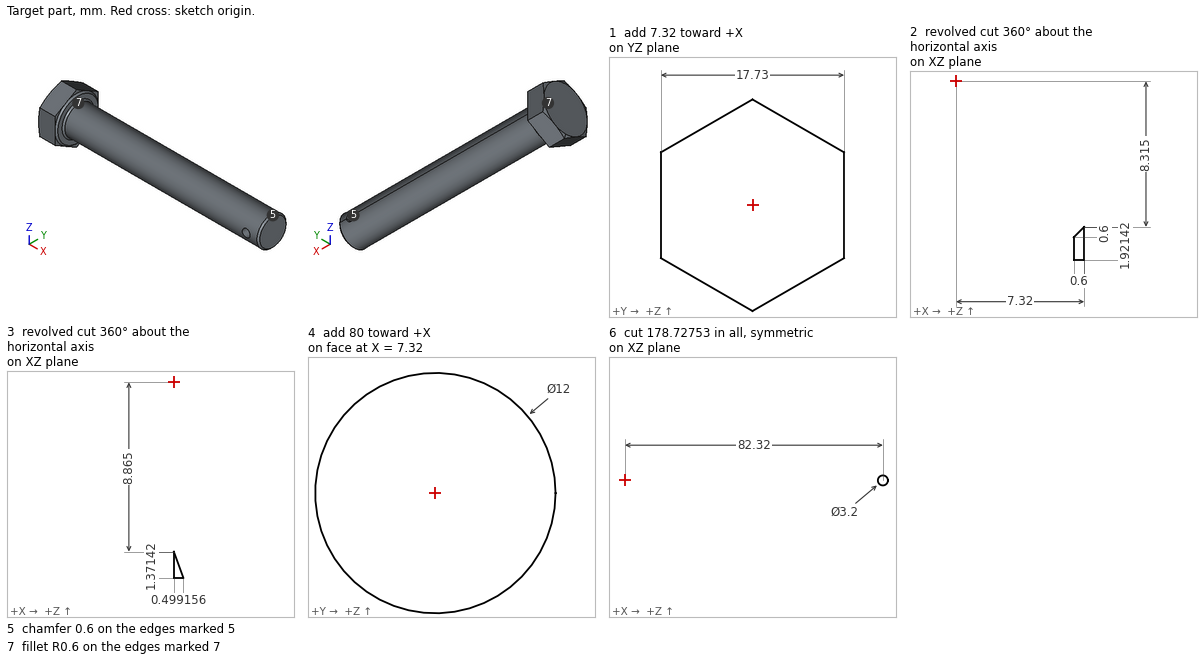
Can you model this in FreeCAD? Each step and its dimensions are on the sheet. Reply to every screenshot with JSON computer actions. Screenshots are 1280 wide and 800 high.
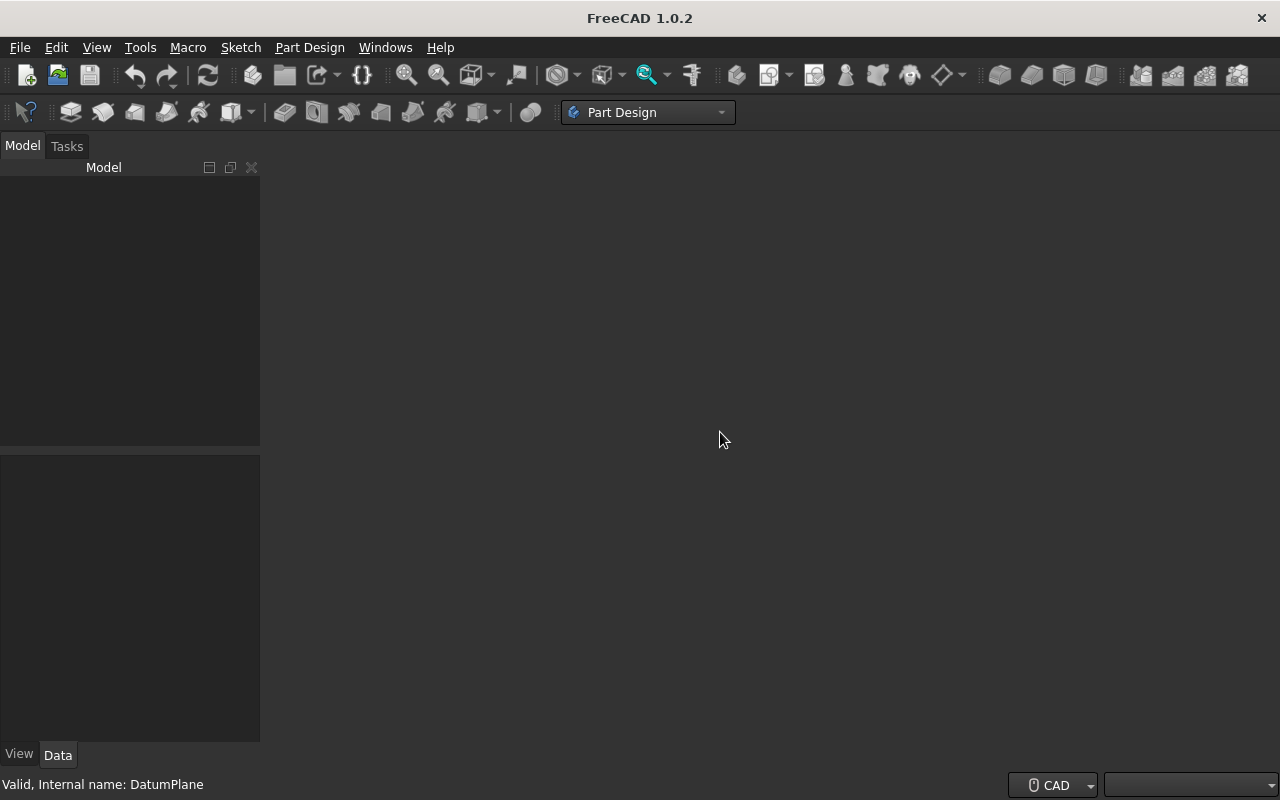
{"action": "left_click", "coordinate": [26, 76]}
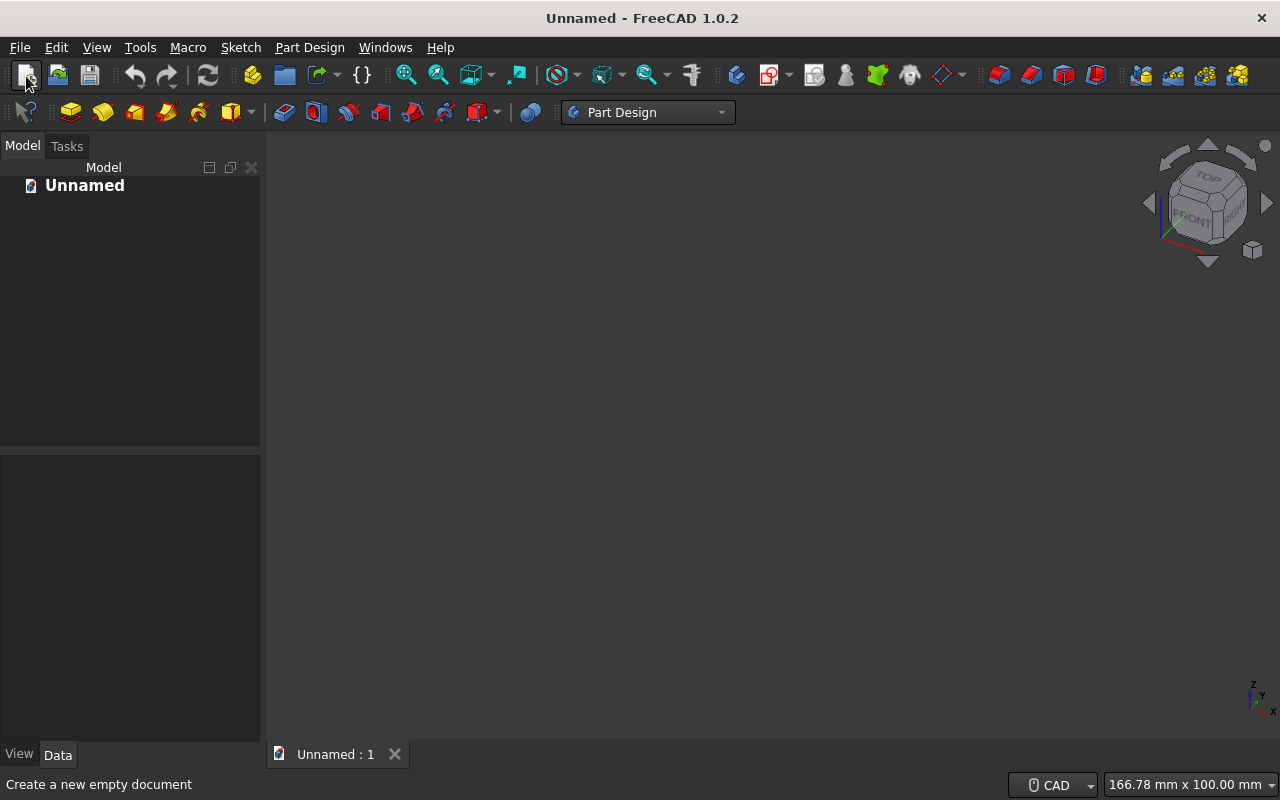
{"action": "left_click", "coordinate": [770, 76]}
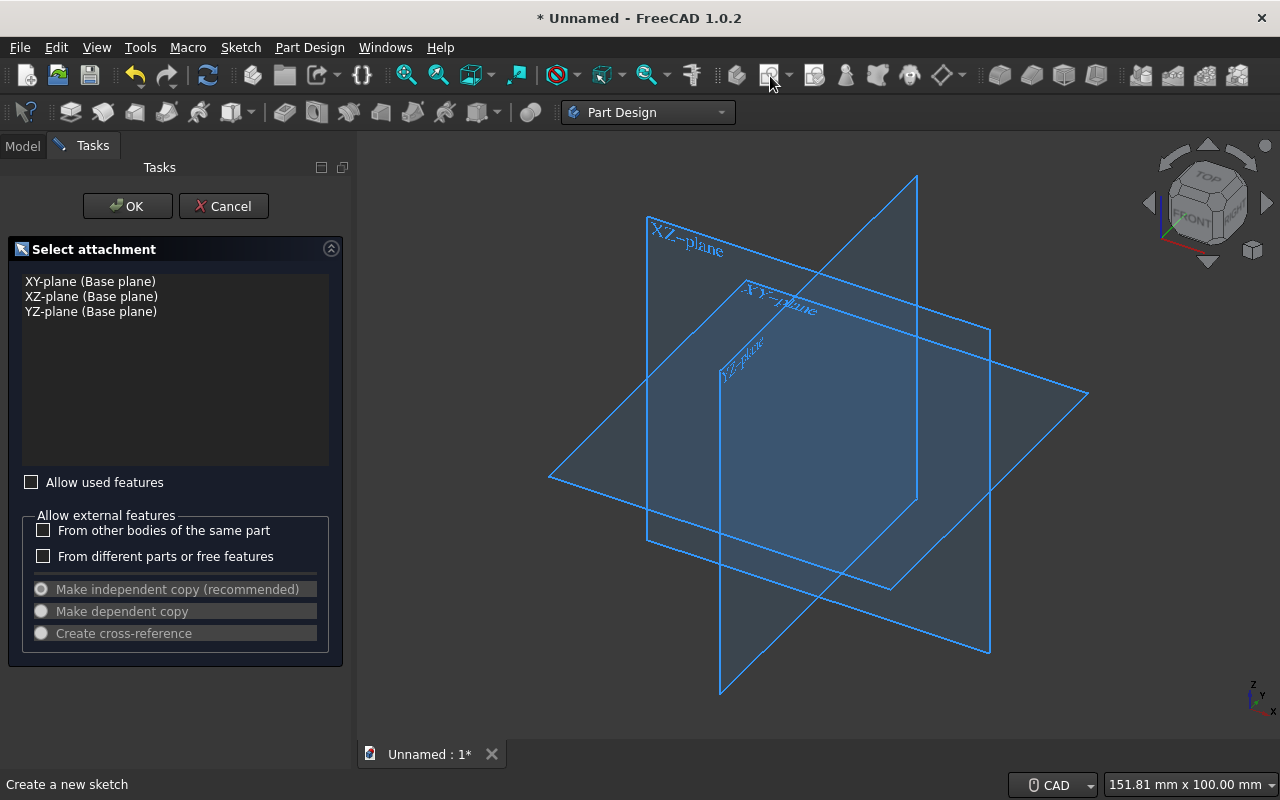
{"action": "left_click", "coordinate": [82, 312]}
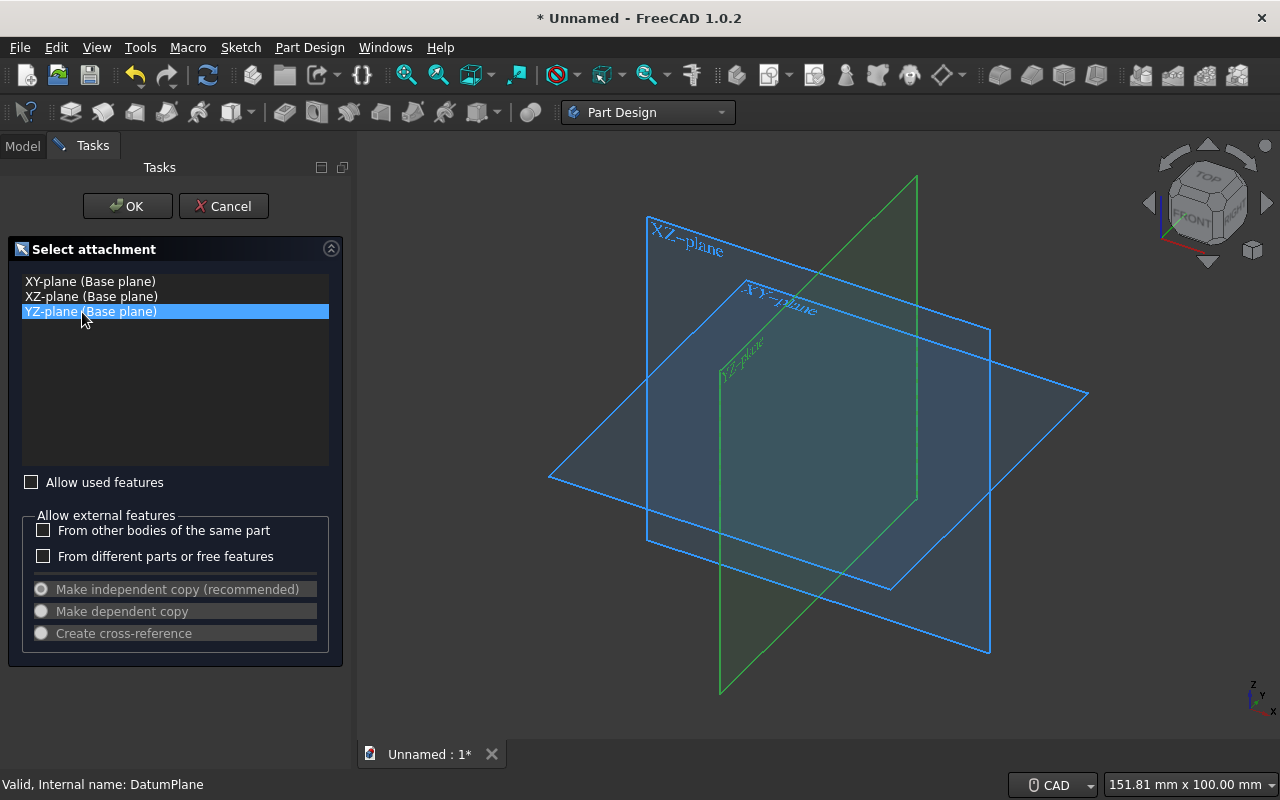
{"action": "left_click", "coordinate": [128, 206]}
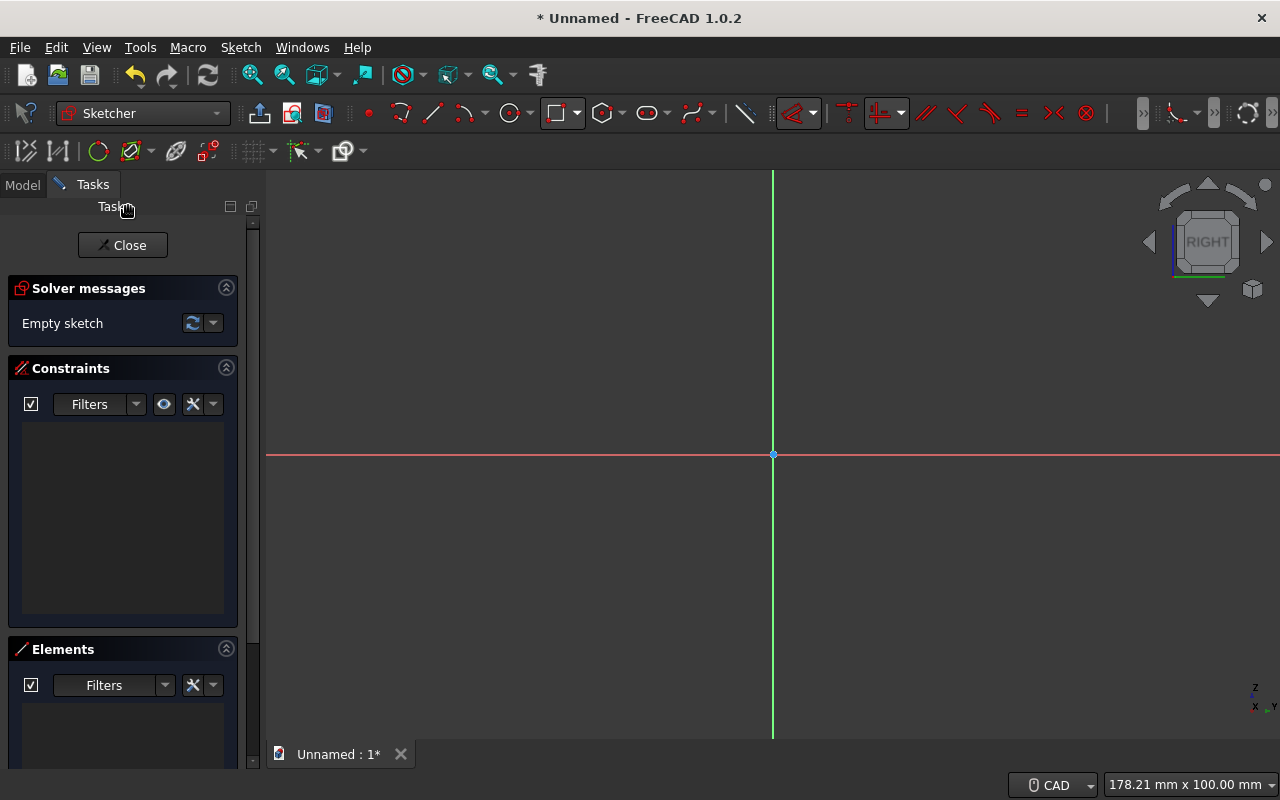
{"action": "scroll", "coordinate": [803, 455], "scroll_direction": "up", "scroll_amount": 6}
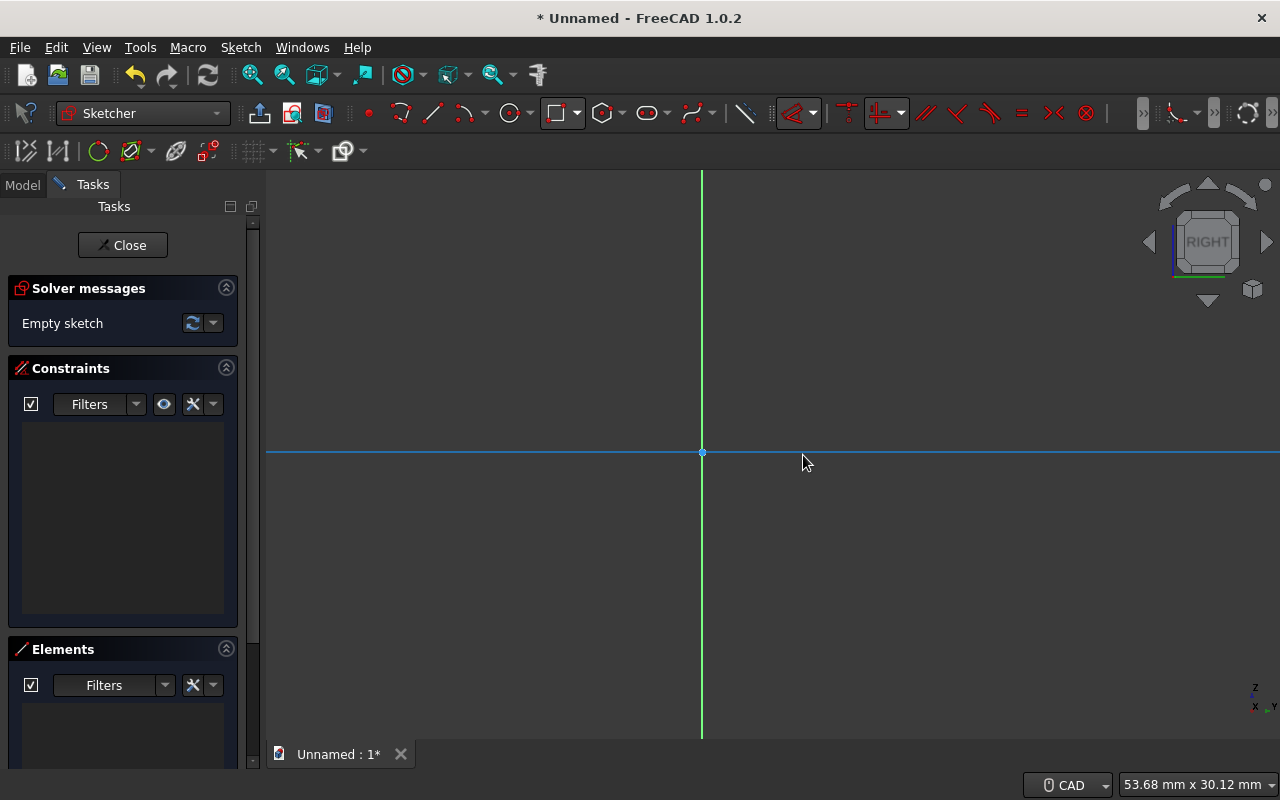
{"action": "key", "text": "g p 6"}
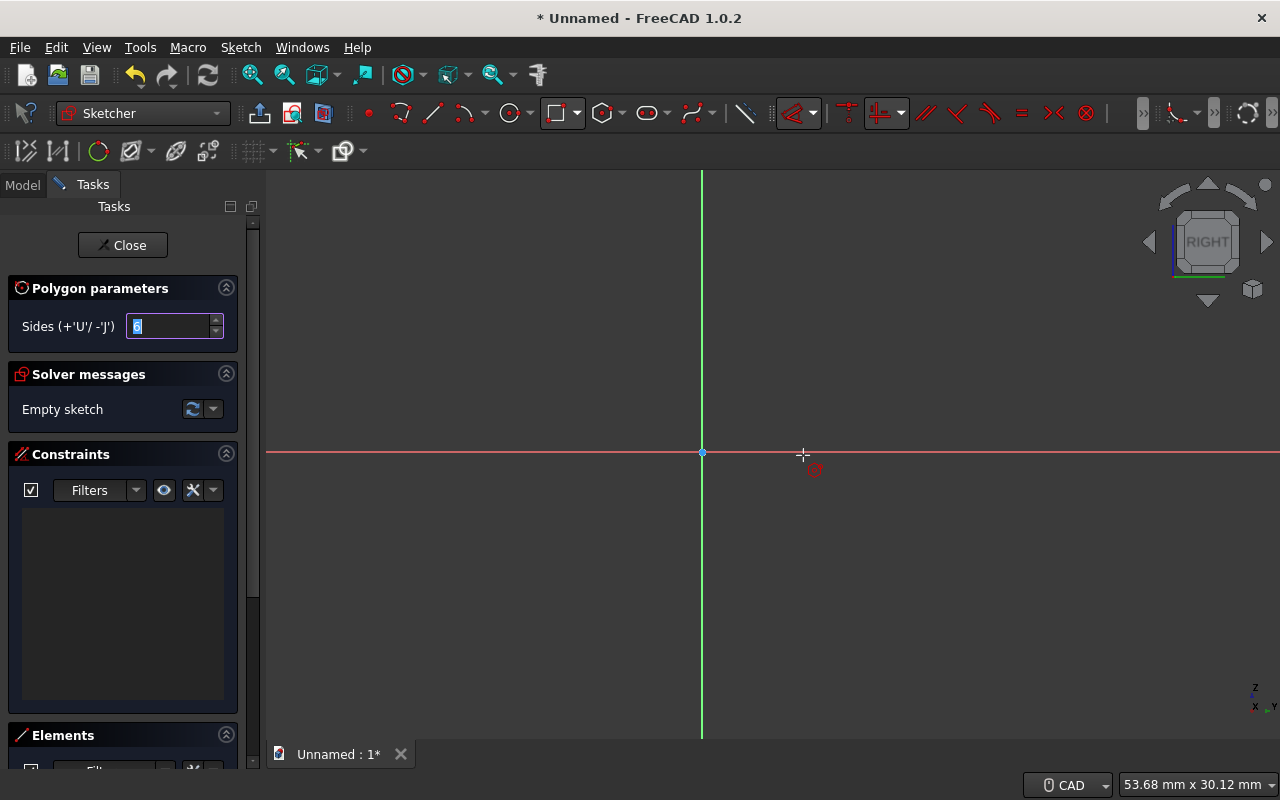
{"action": "left_click", "coordinate": [702, 452]}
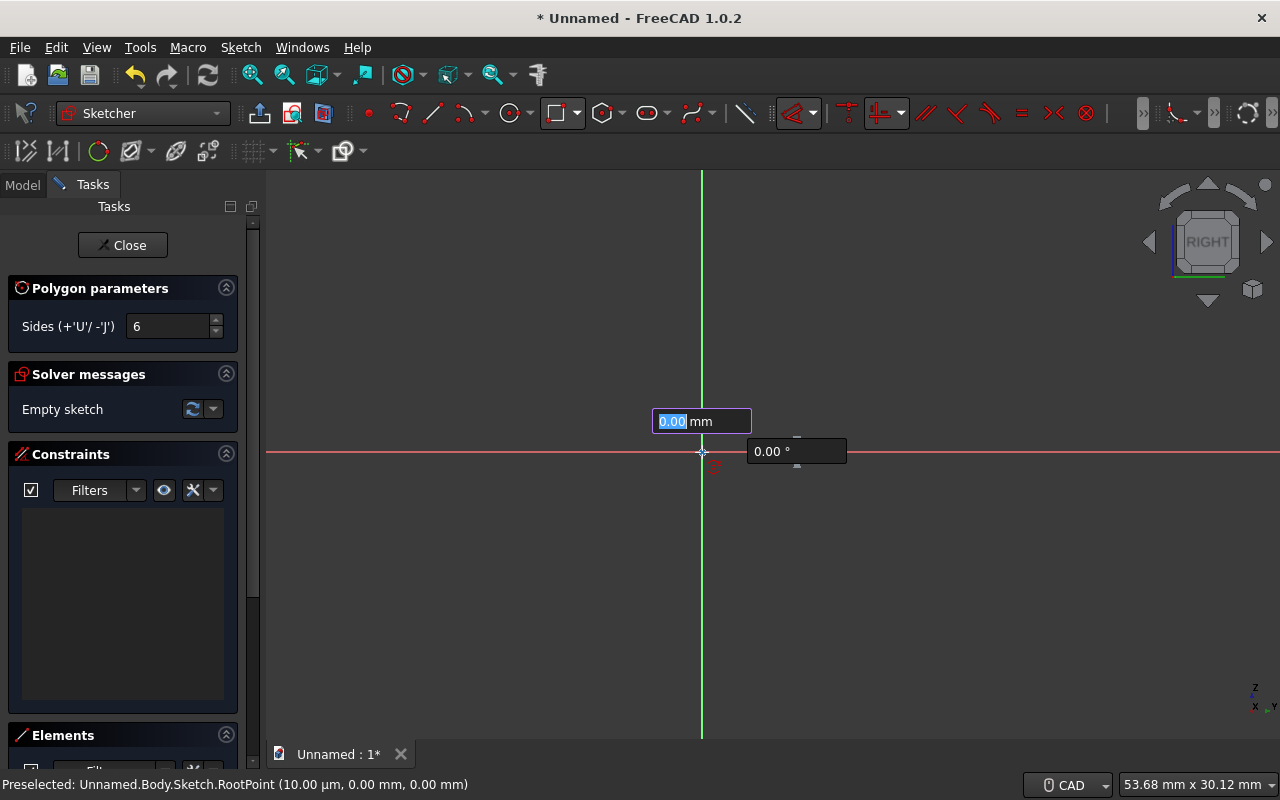
{"action": "left_click", "coordinate": [702, 646]}
{"action": "right_click", "coordinate": [702, 646]}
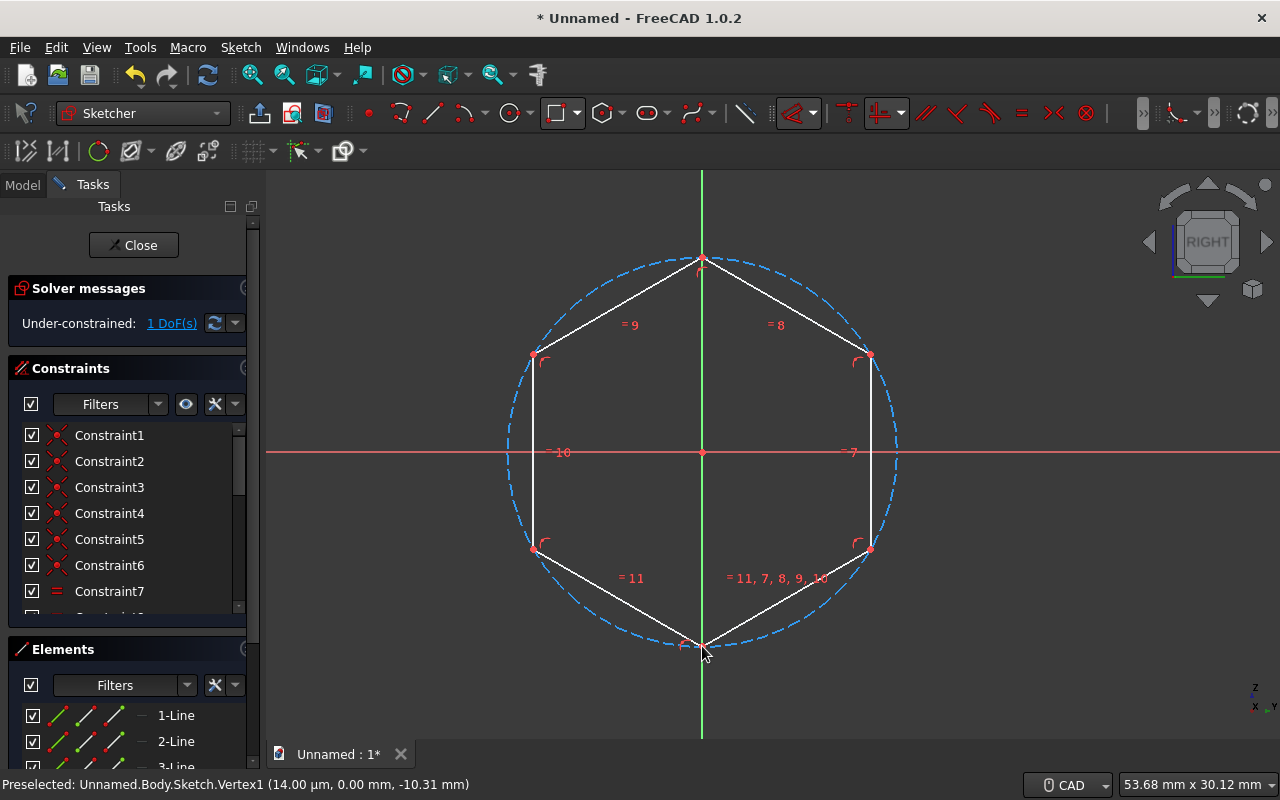
{"action": "left_click", "coordinate": [533, 355]}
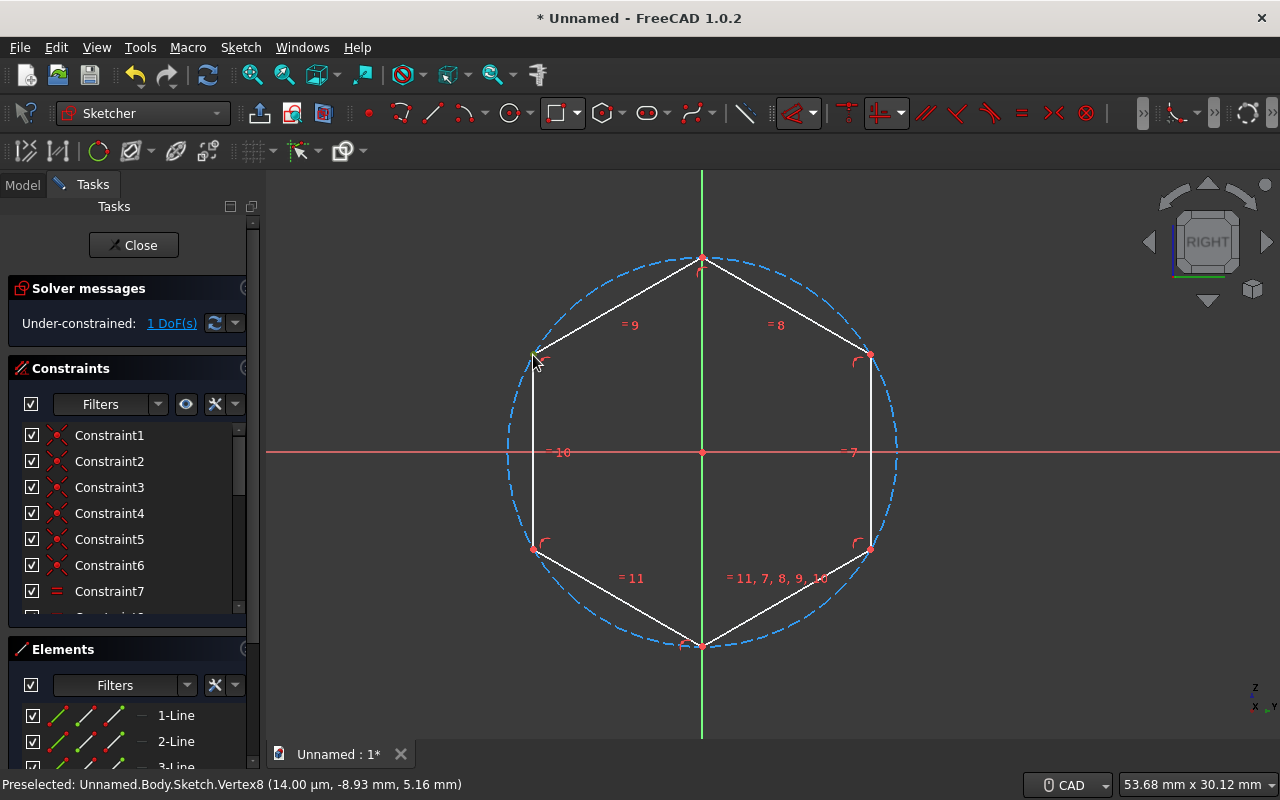
{"action": "left_click", "coordinate": [871, 550]}